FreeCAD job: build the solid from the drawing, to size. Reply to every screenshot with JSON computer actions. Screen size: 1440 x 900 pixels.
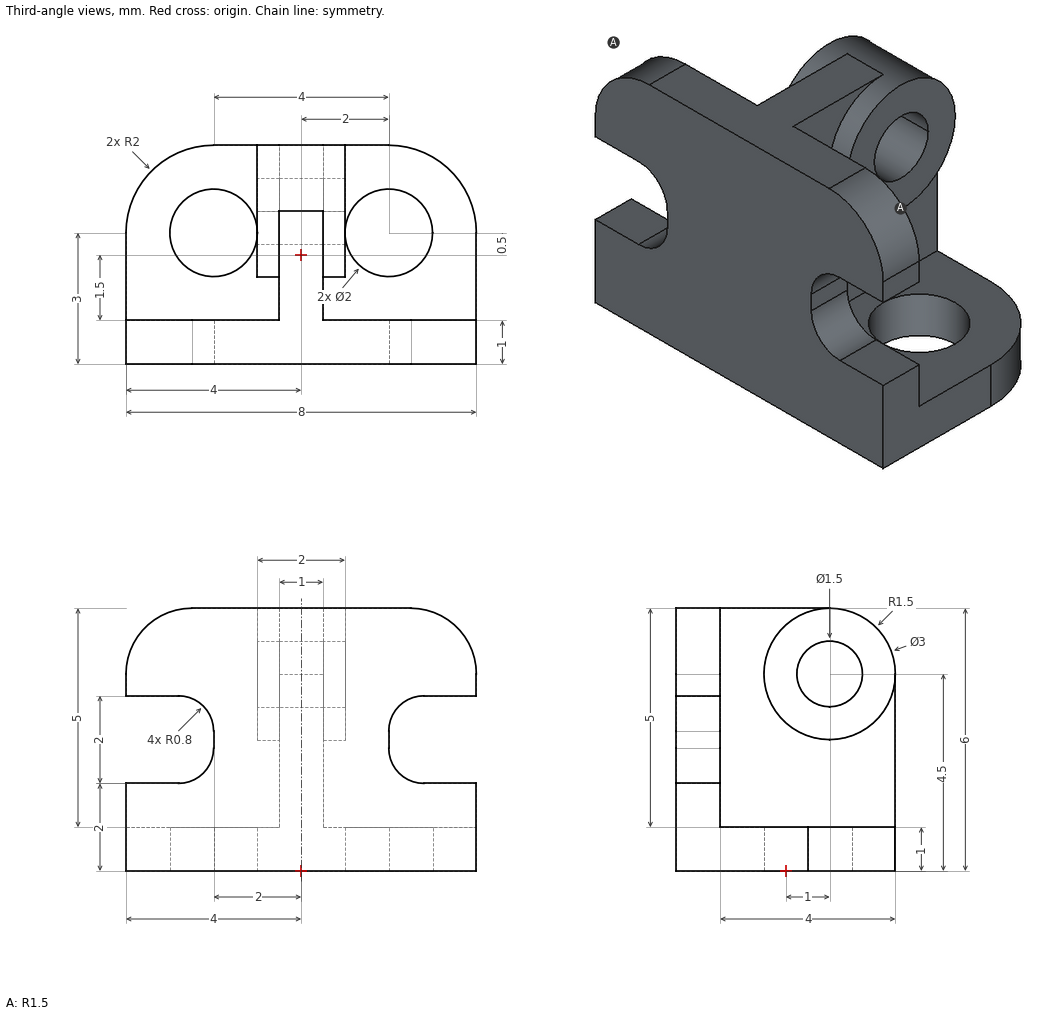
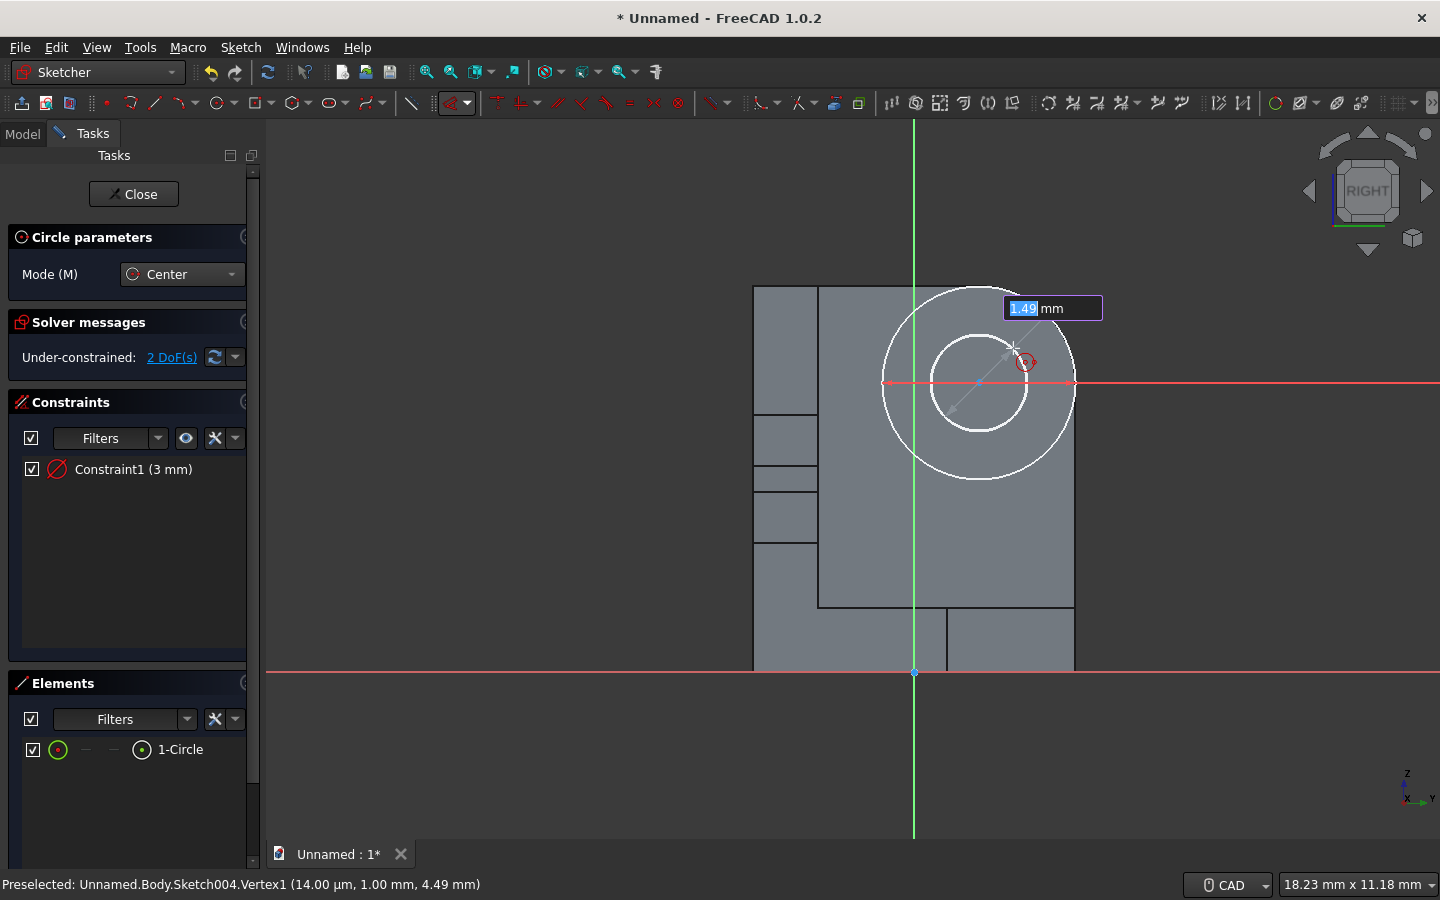
{"action": "type", "text": "1.5"}
{"action": "key", "text": "Return"}
{"action": "key", "text": "Escape"}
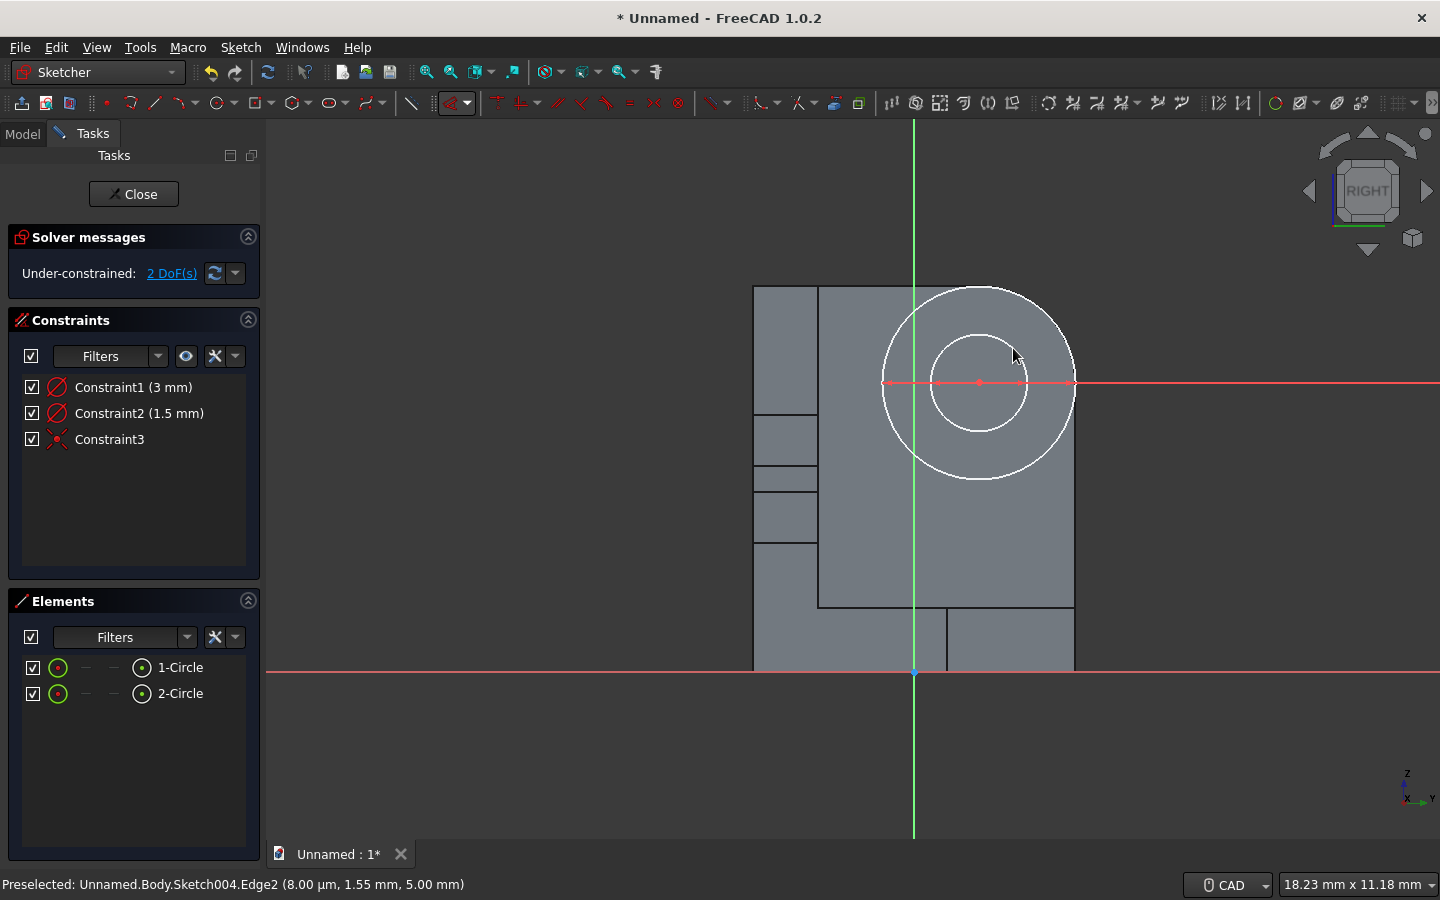
{"action": "left_click", "coordinate": [979, 383]}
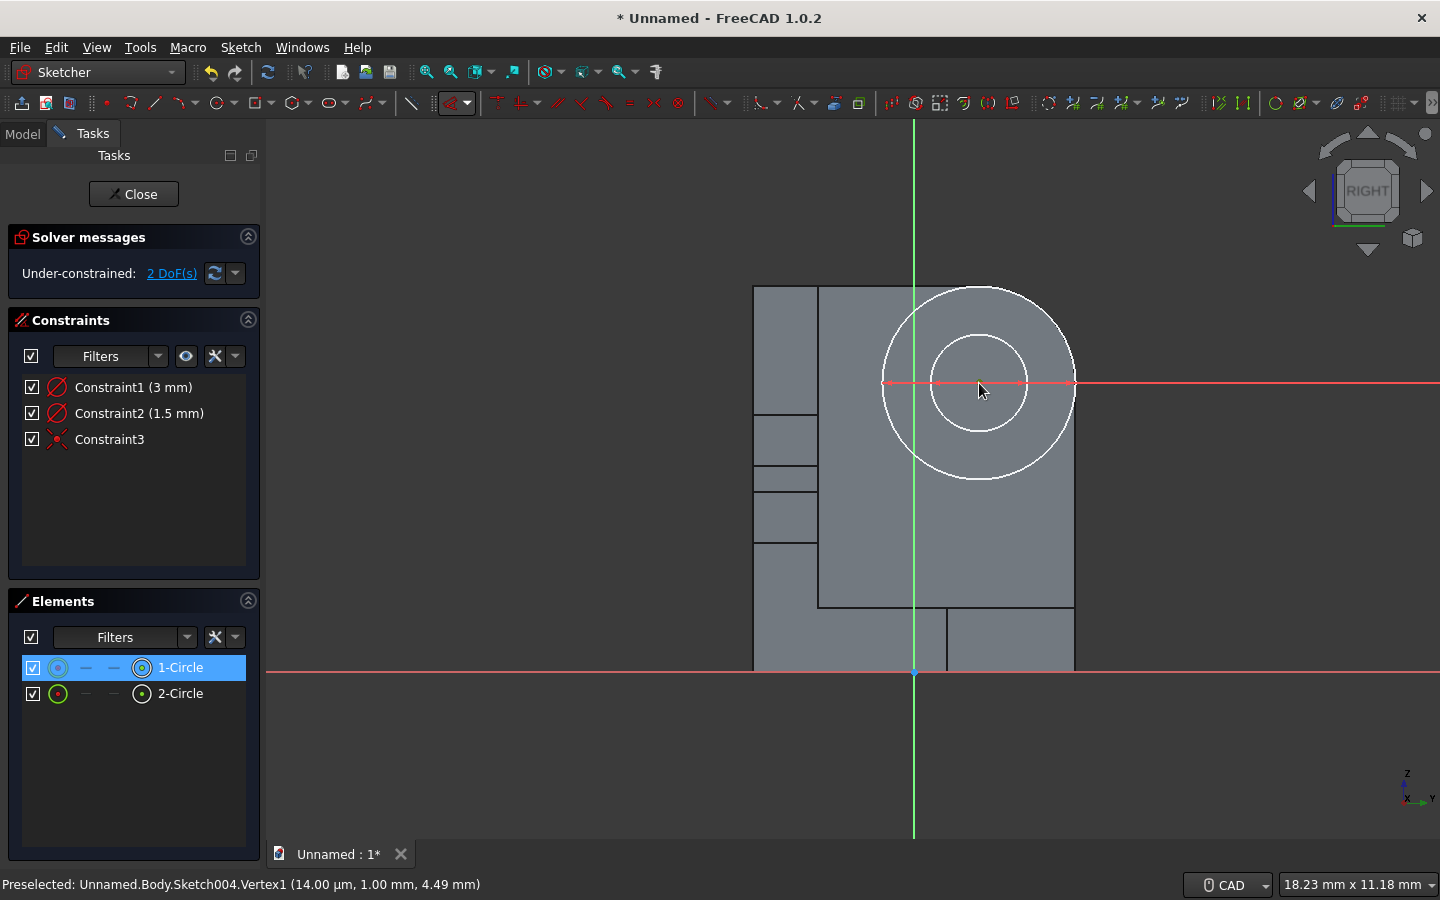
{"action": "left_click", "coordinate": [470, 104]}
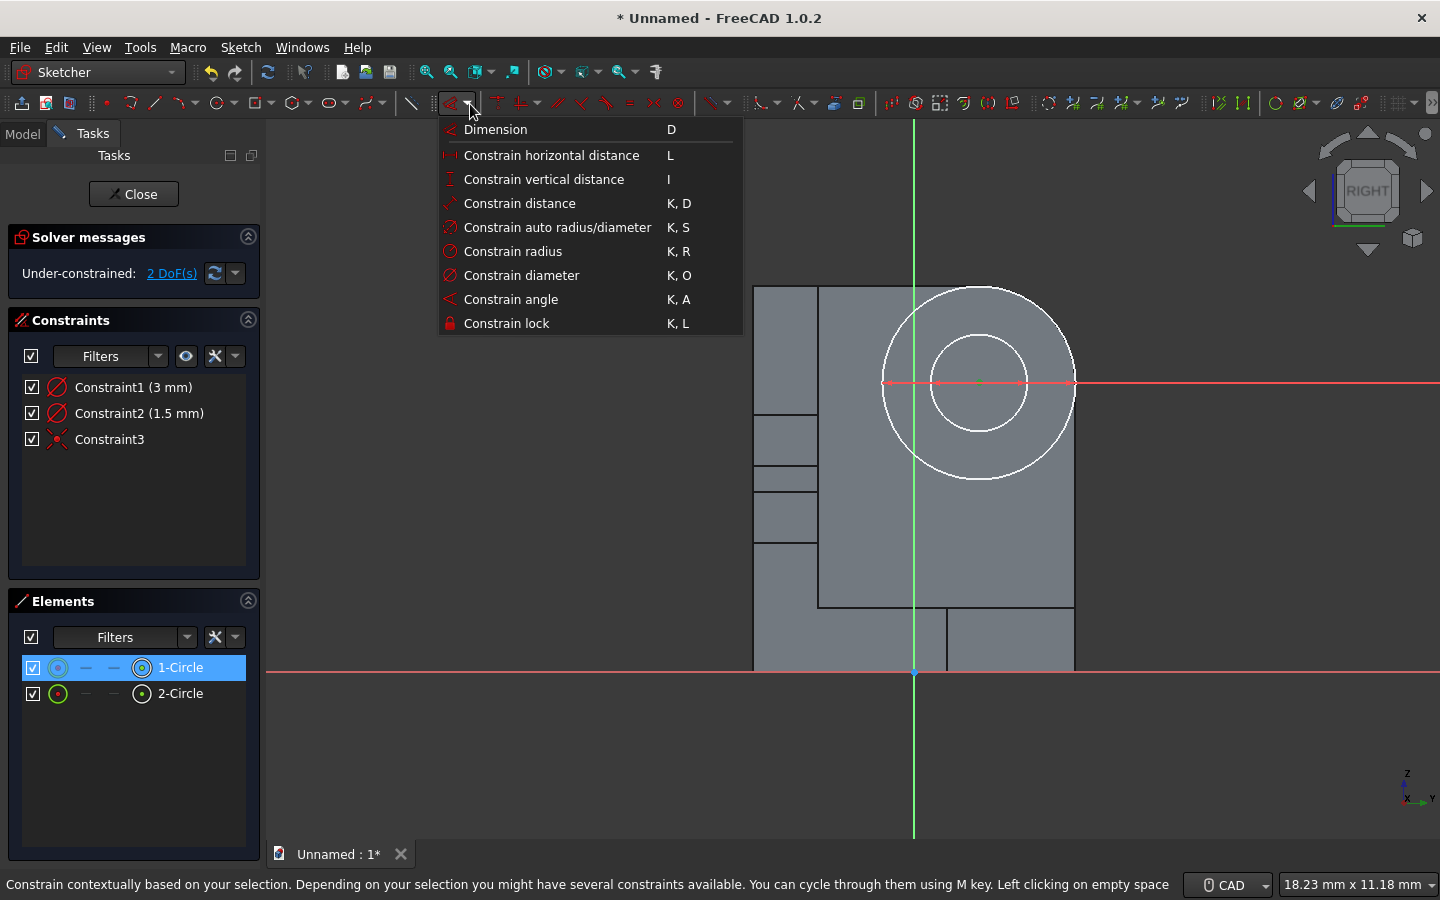
{"action": "left_click", "coordinate": [591, 155]}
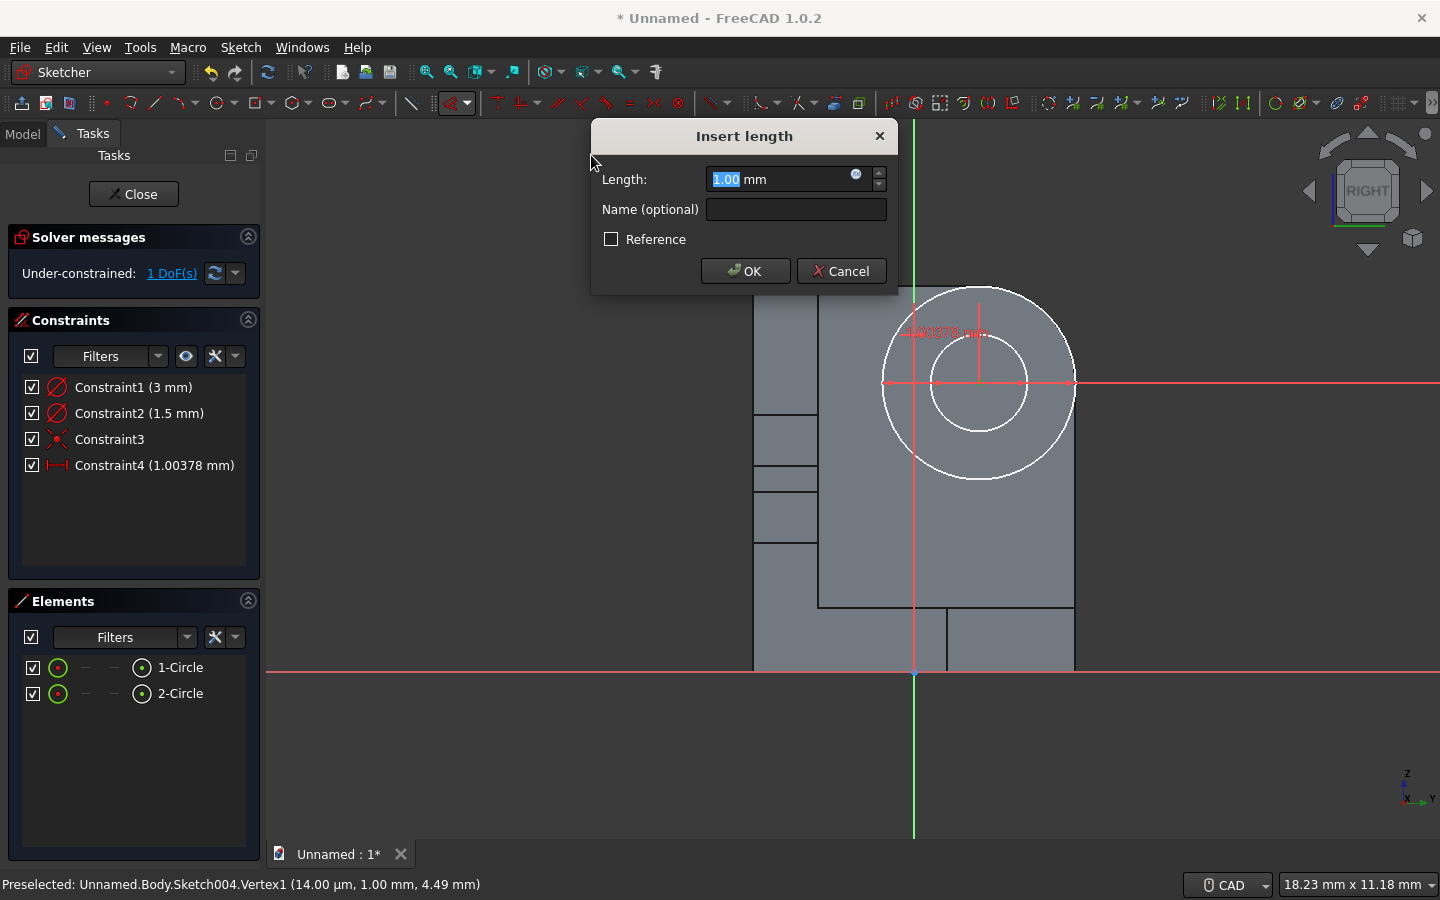
{"action": "type", "text": "1"}
{"action": "key", "text": "Return"}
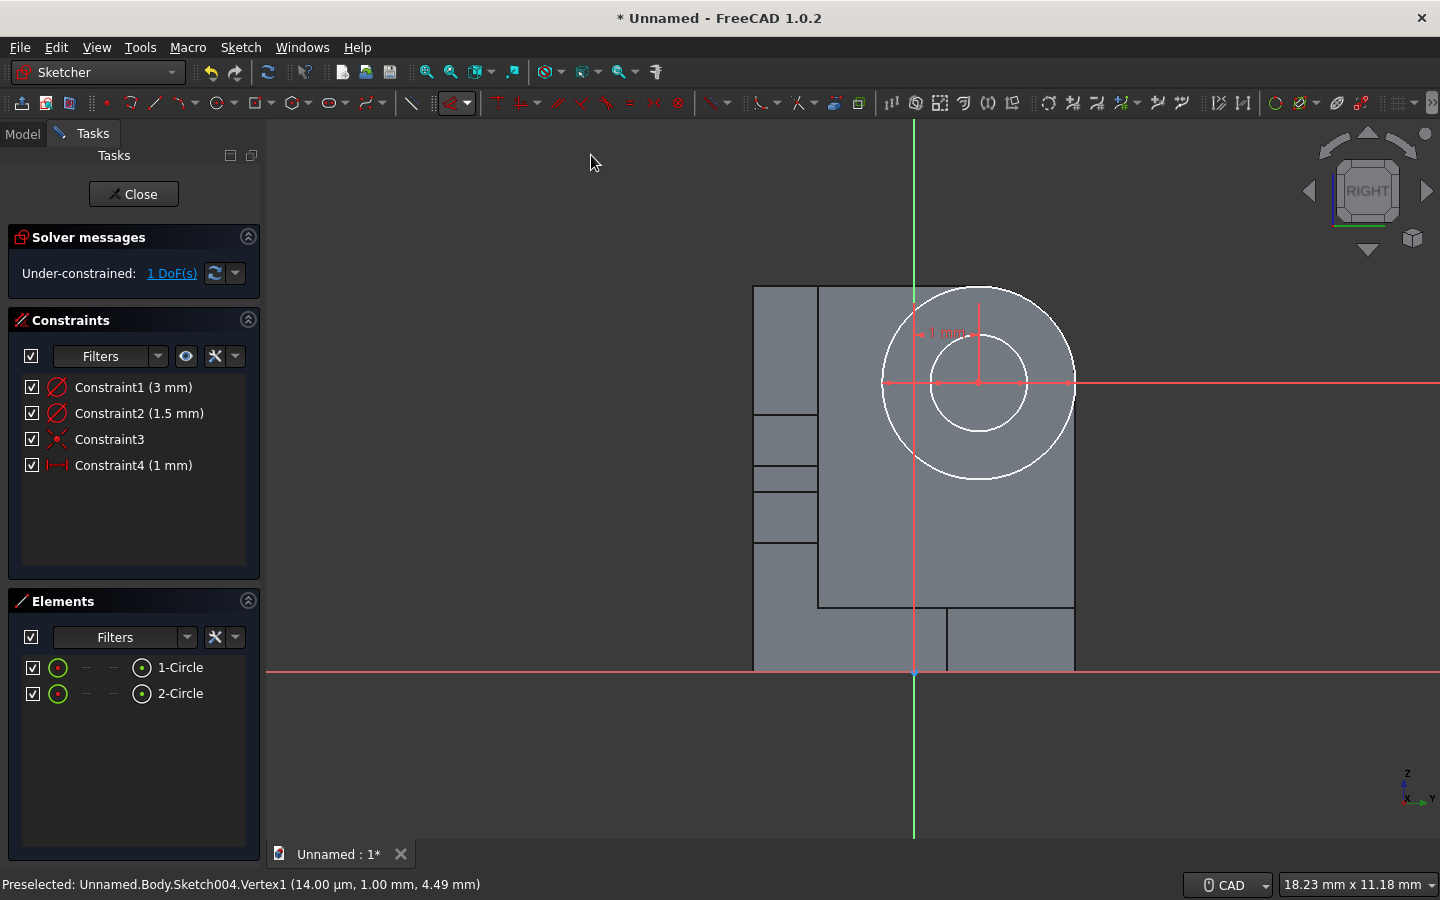
{"action": "left_click", "coordinate": [979, 383]}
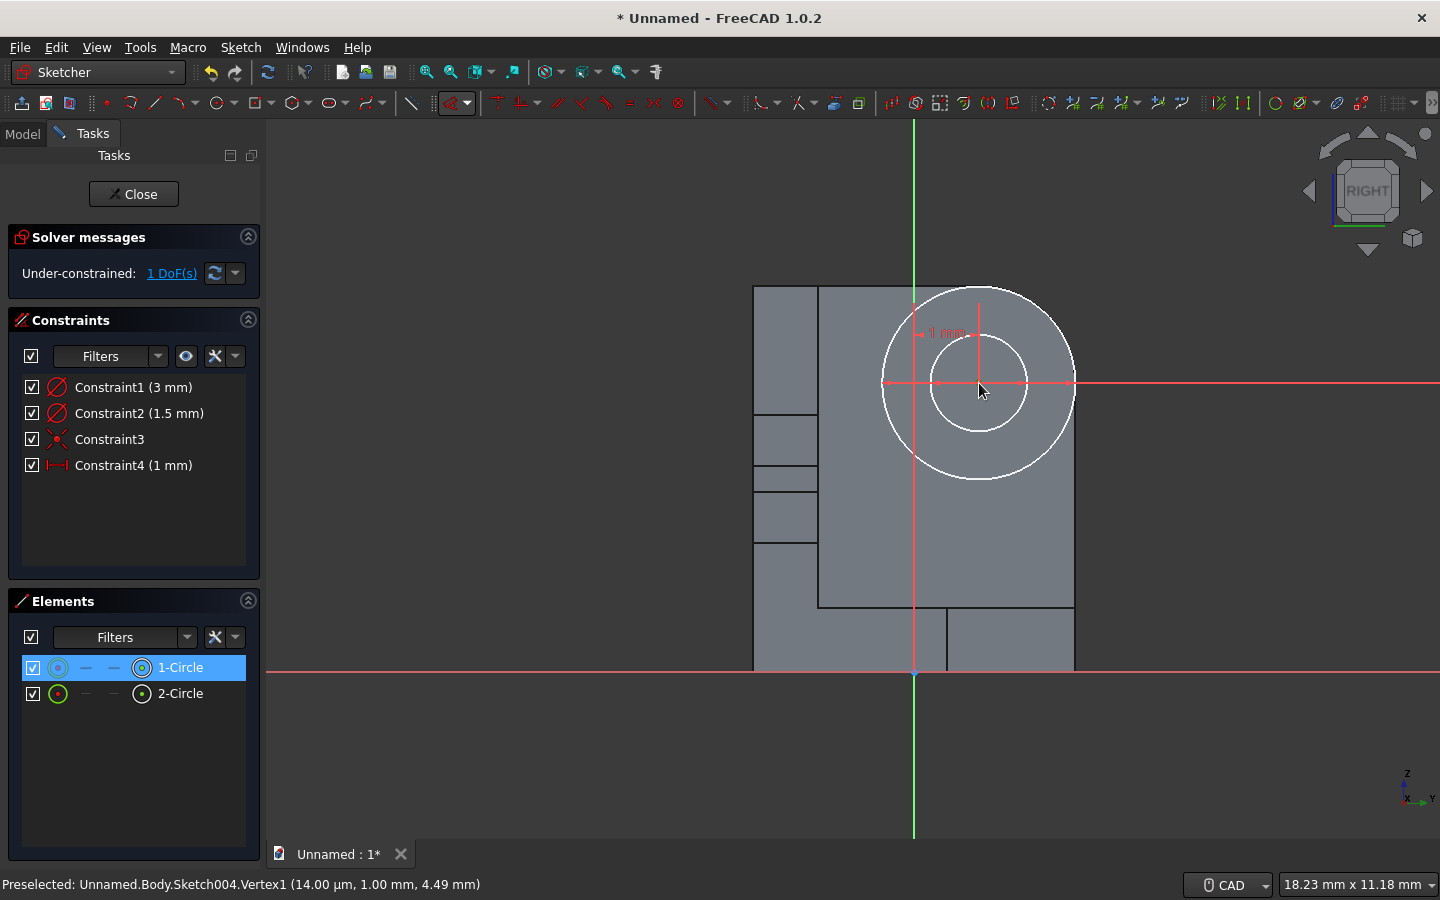
{"action": "key", "text": "i"}